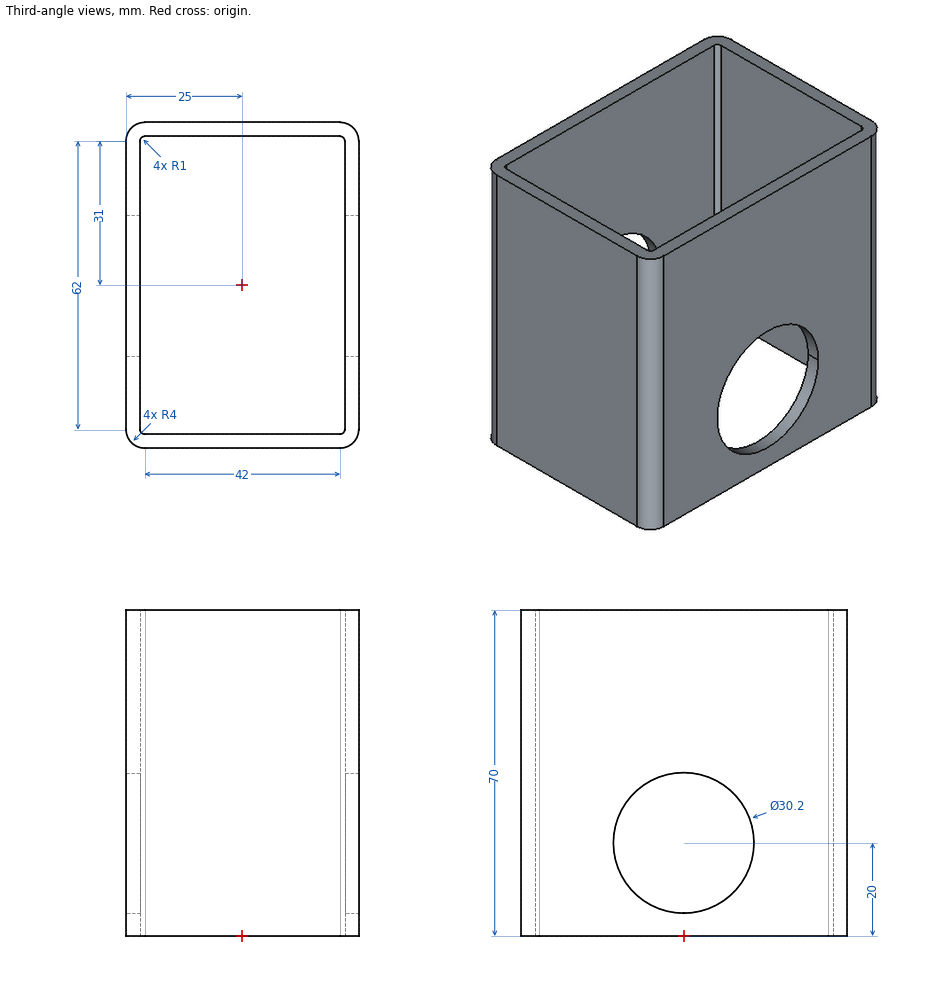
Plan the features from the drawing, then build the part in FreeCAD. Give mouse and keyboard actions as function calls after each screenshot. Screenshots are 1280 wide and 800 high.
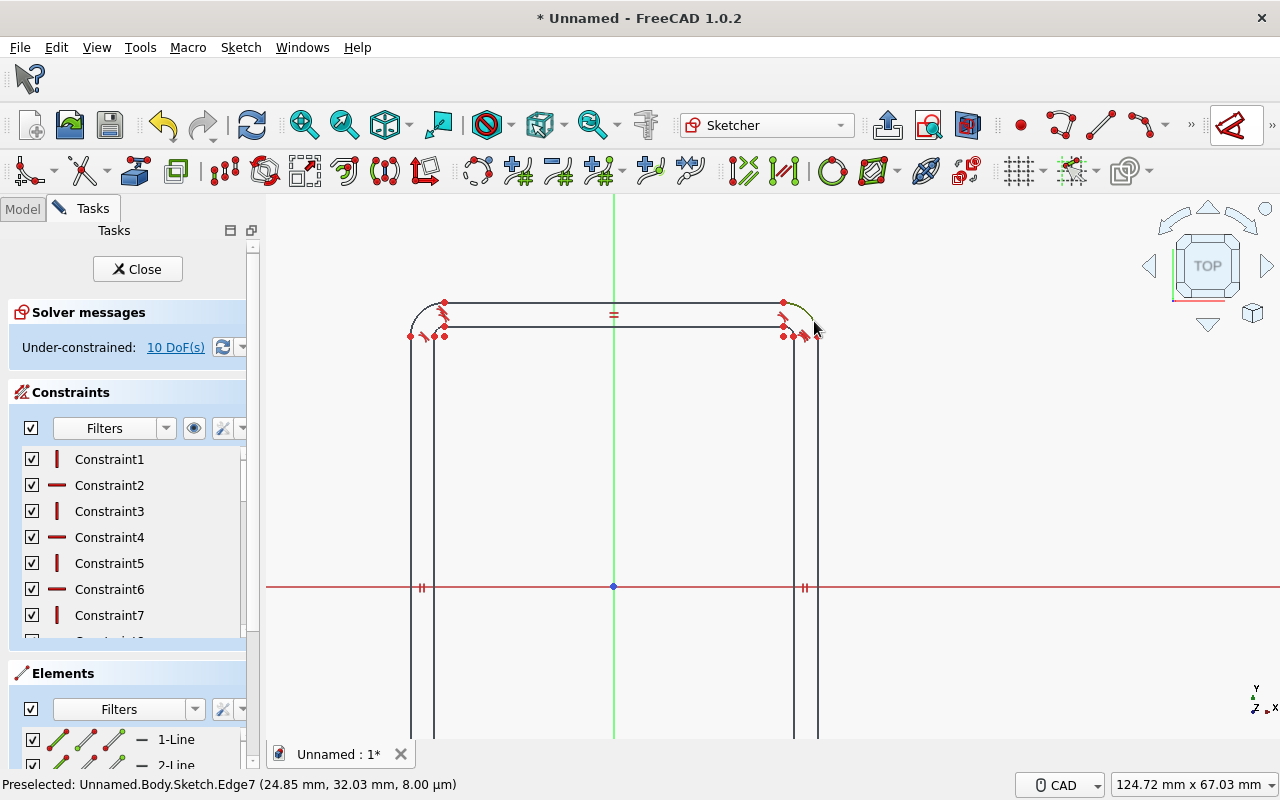
click(429, 307)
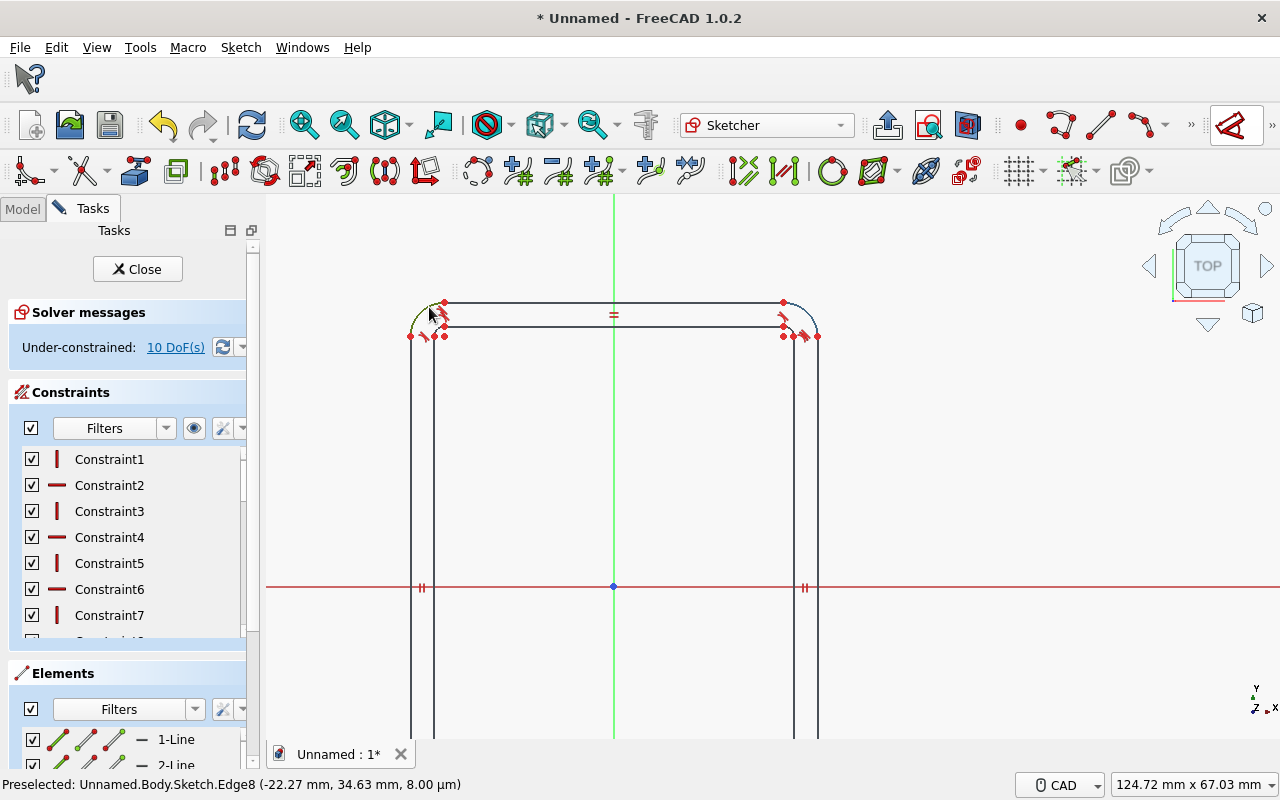
key(e)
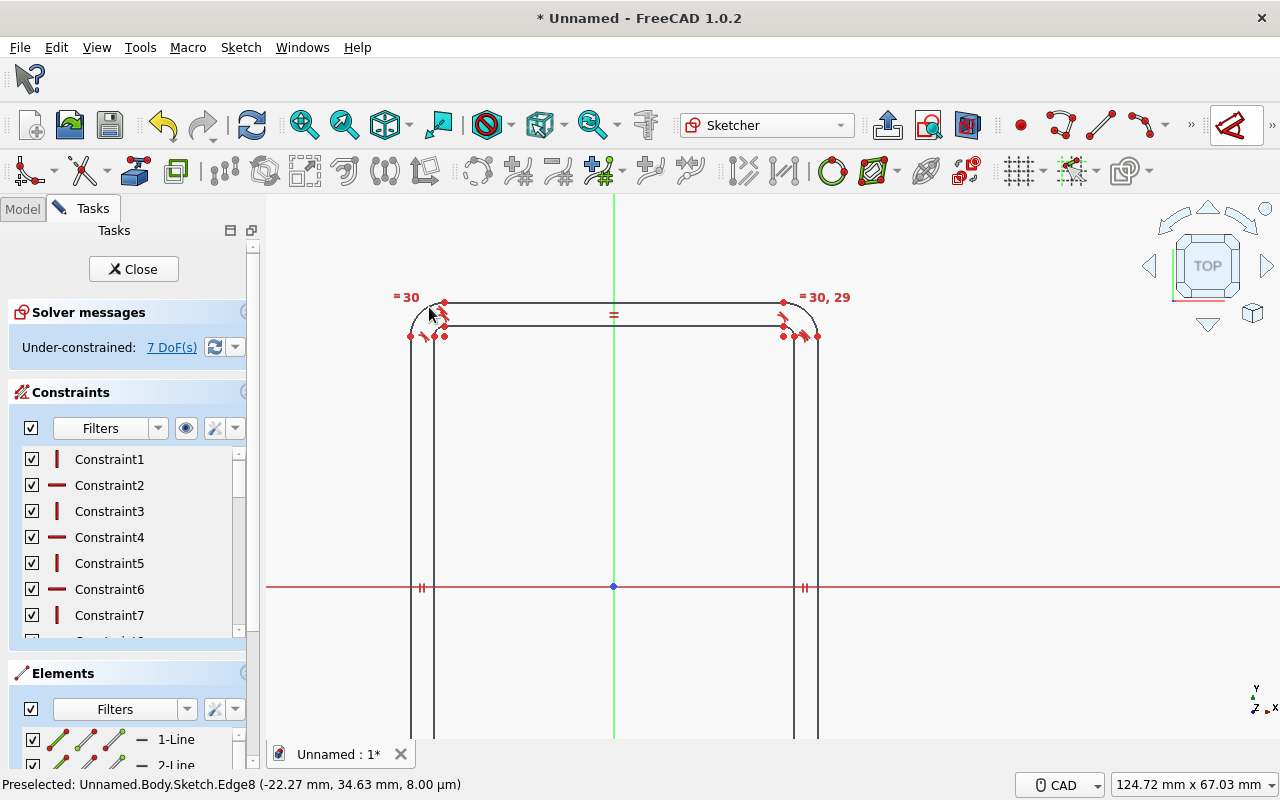
scroll(437, 329, up, 3)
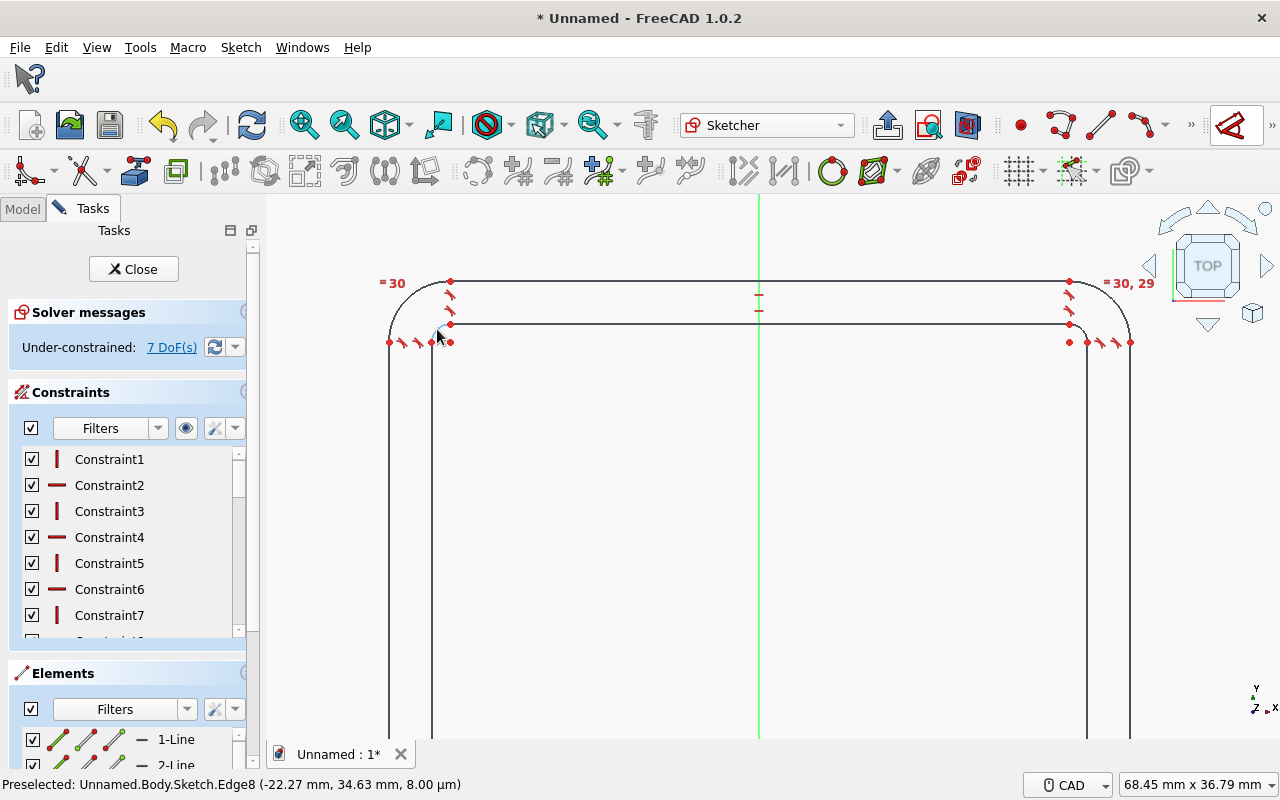
click(437, 330)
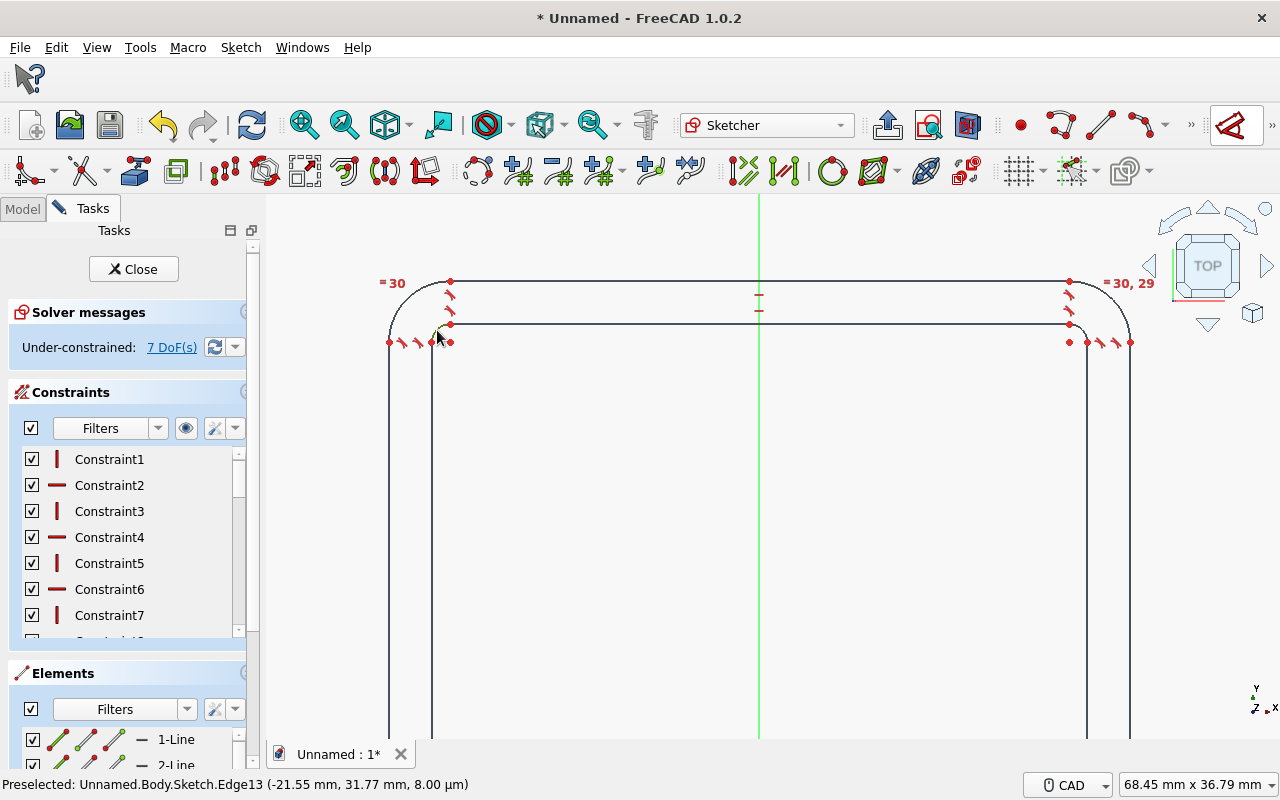
scroll(681, 324, down, 6)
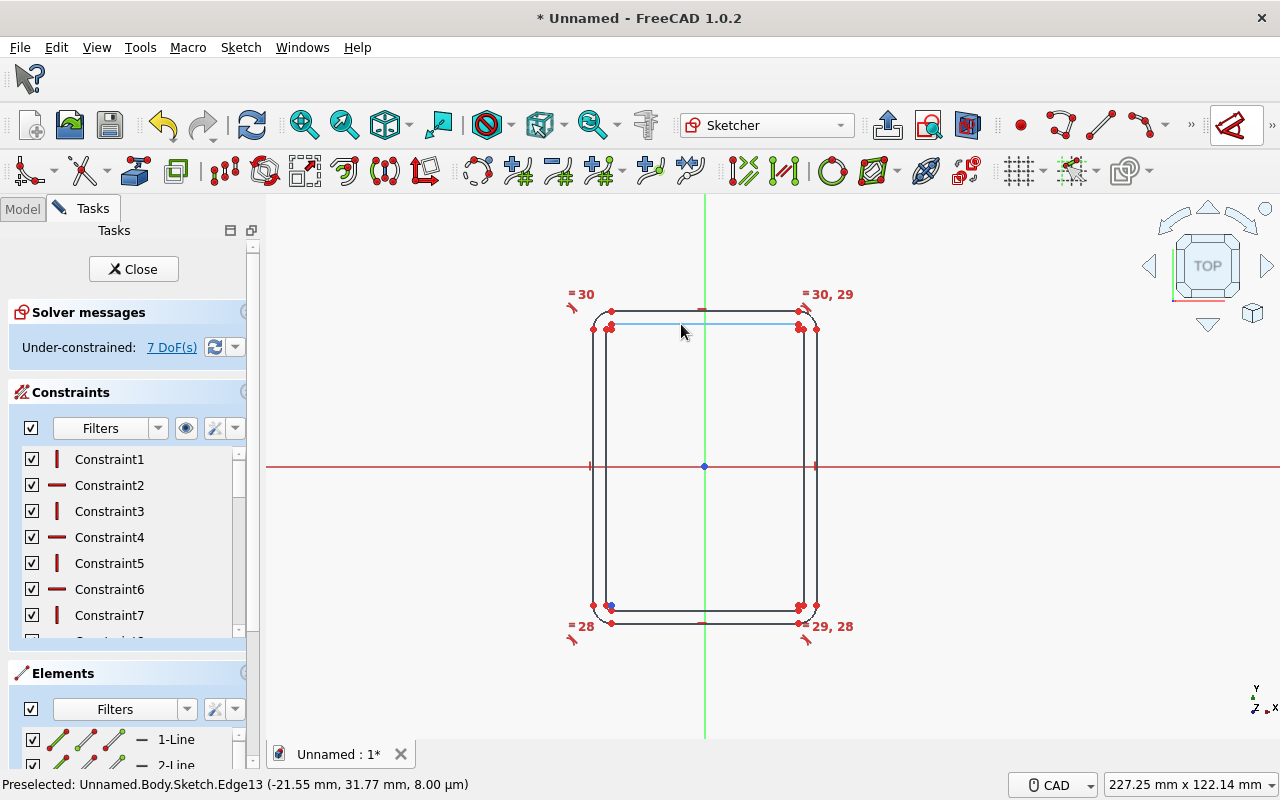
scroll(608, 609, up, 7)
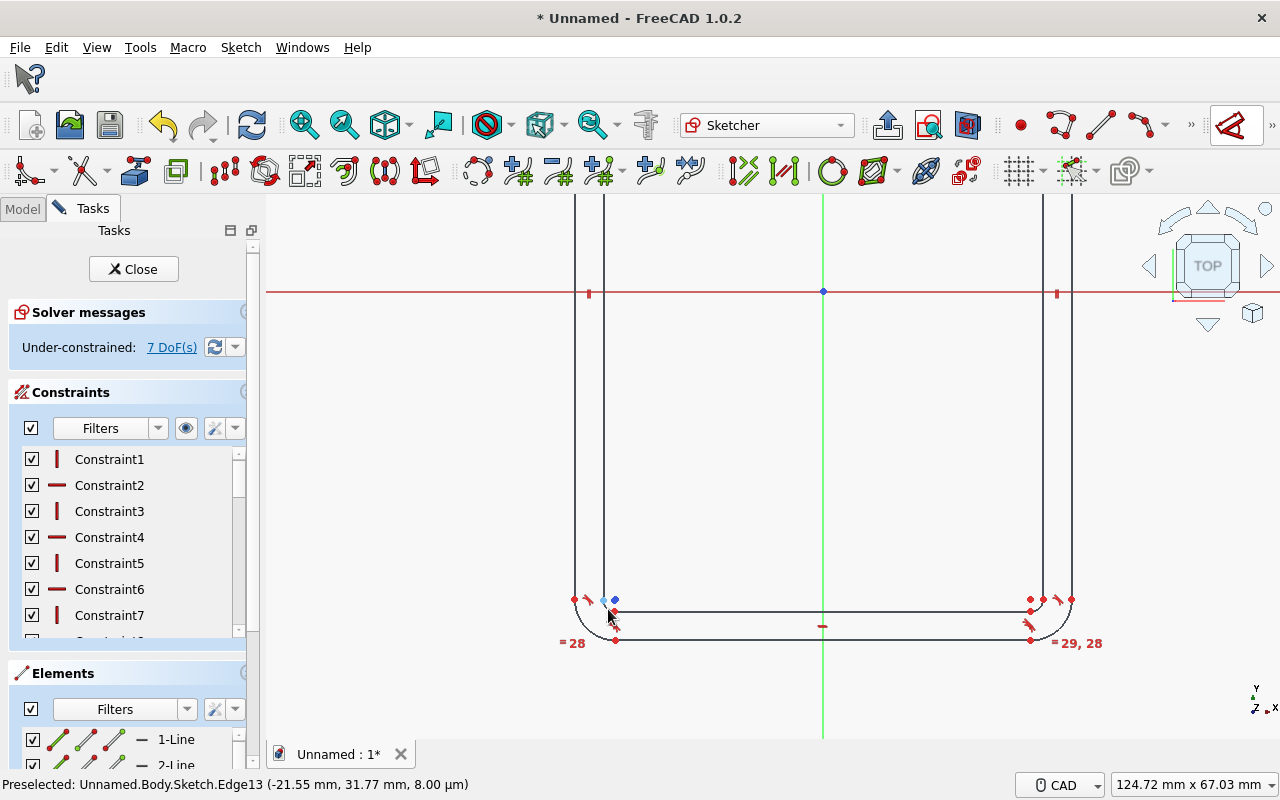
click(606, 608)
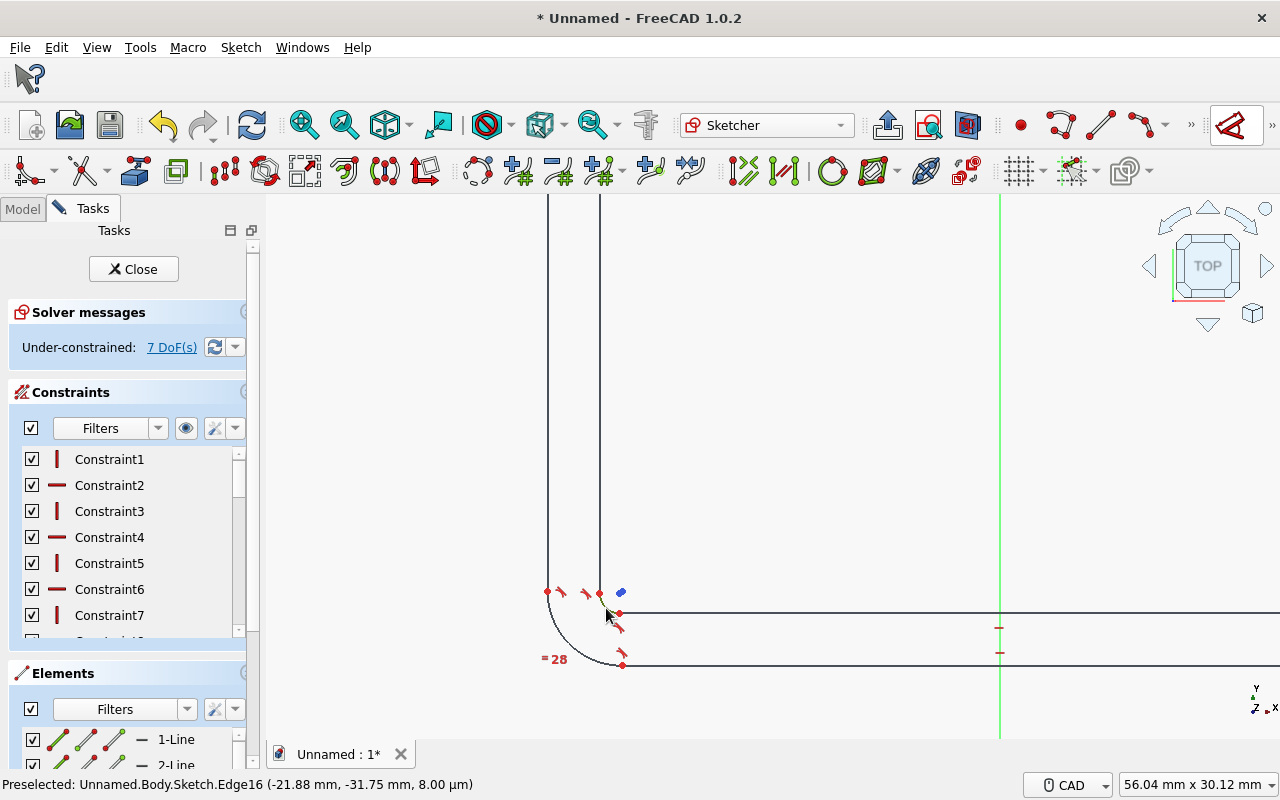
key(e)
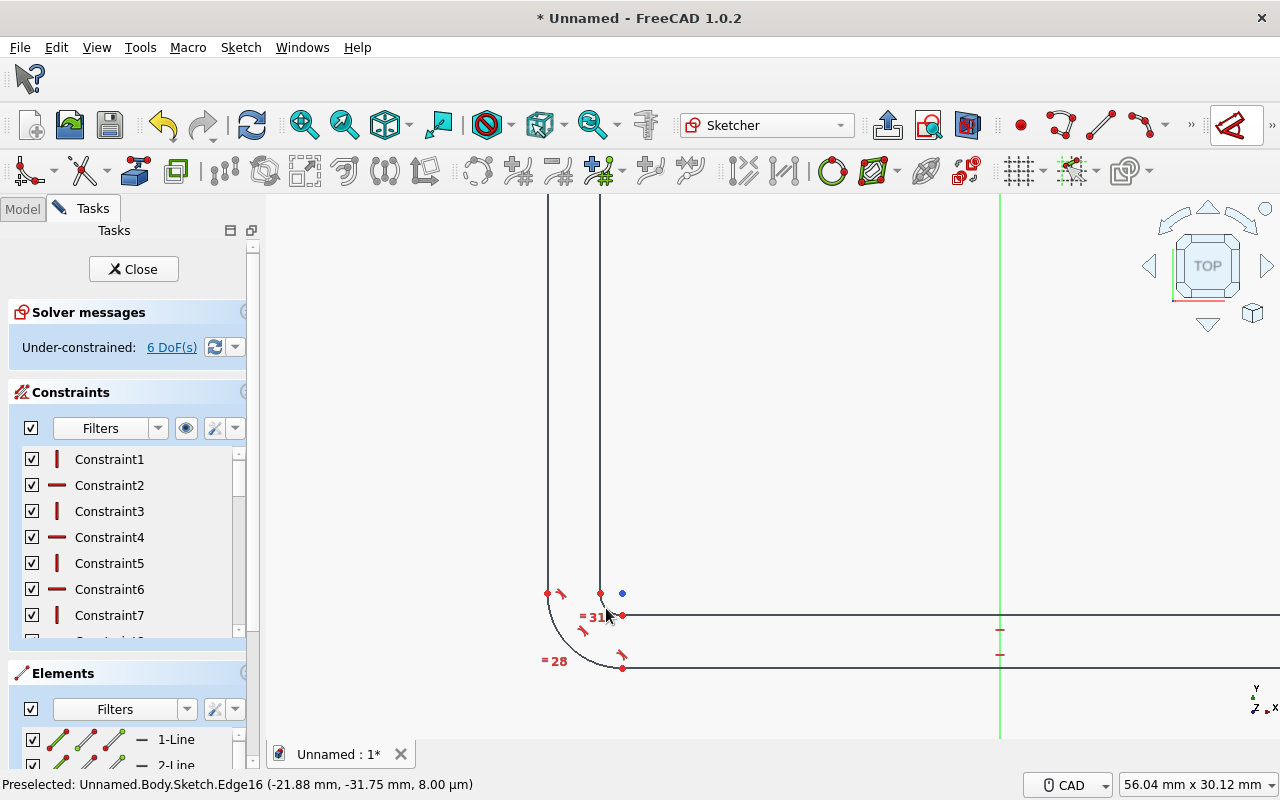
click(1230, 126)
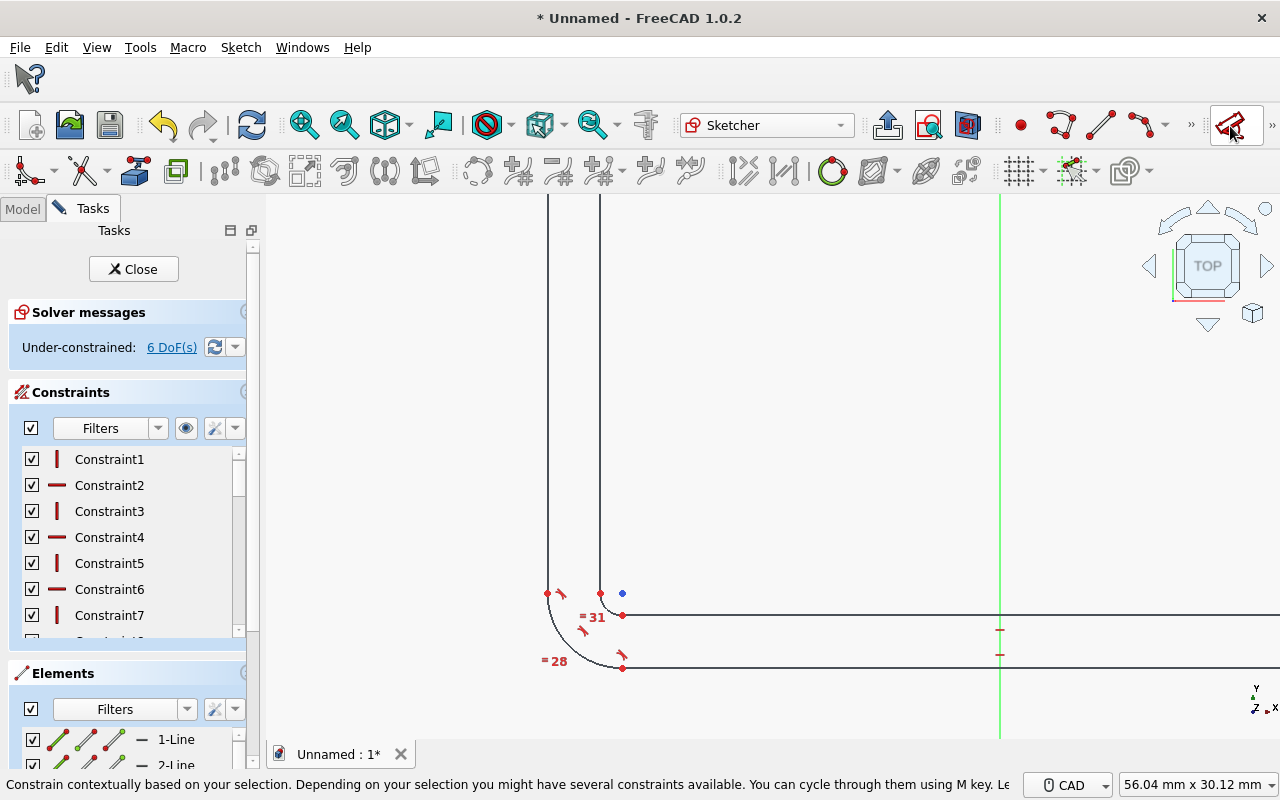
click(556, 627)
click(527, 641)